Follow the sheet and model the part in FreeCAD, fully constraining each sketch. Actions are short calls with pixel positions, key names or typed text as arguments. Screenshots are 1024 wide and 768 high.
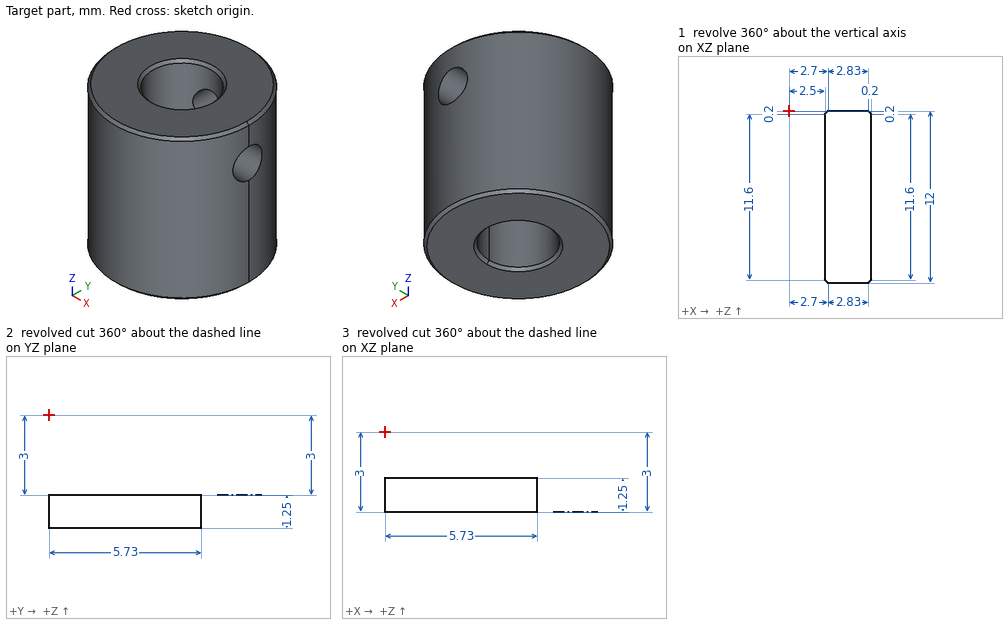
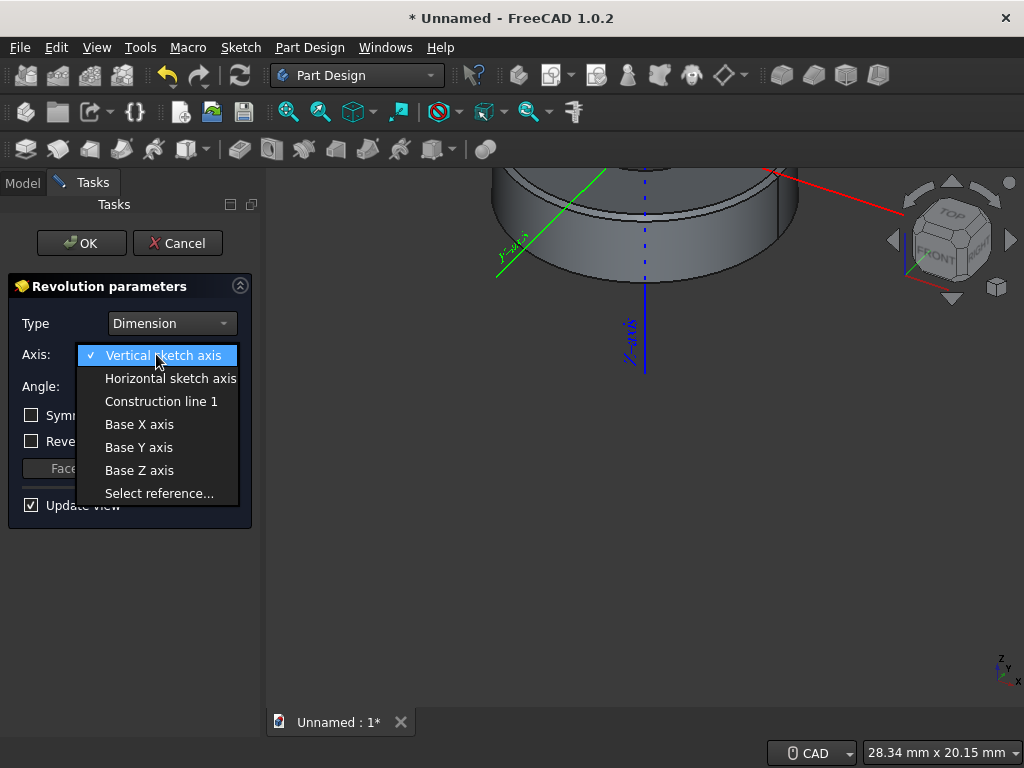
click(156, 402)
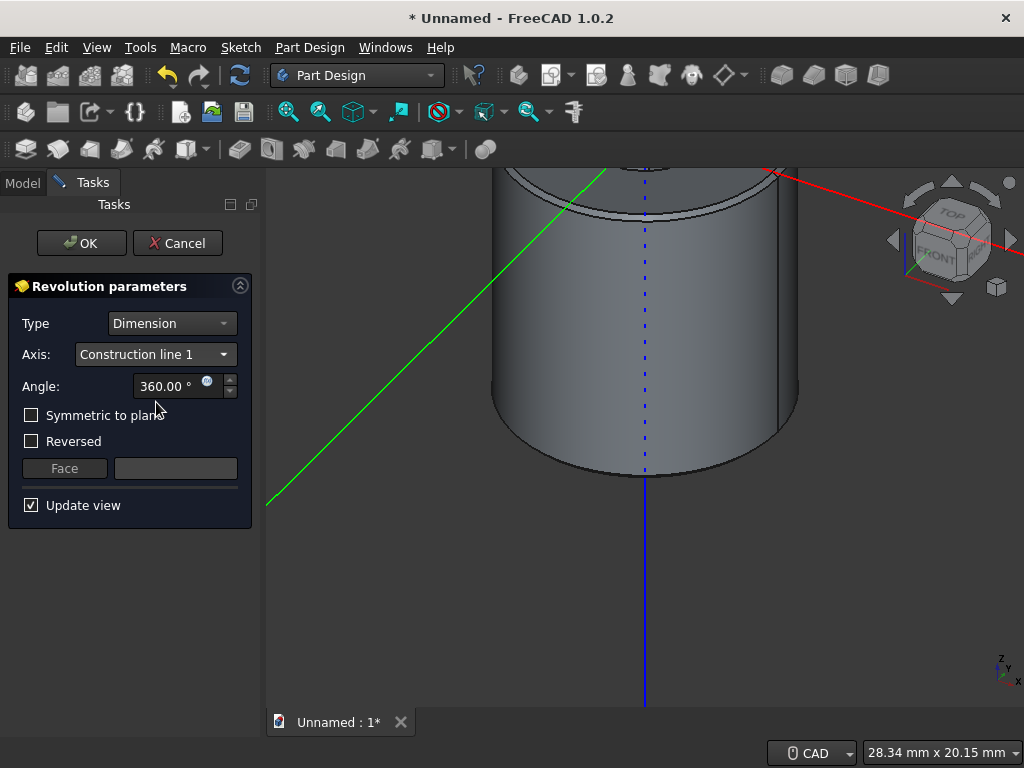
click(82, 243)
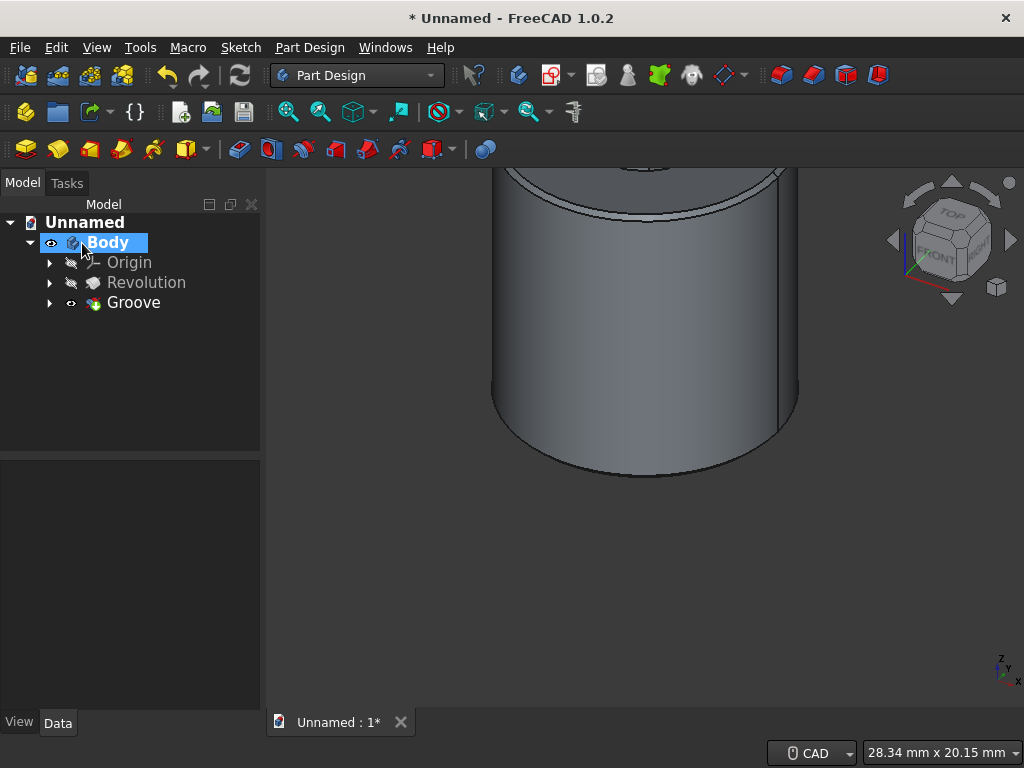
click(290, 112)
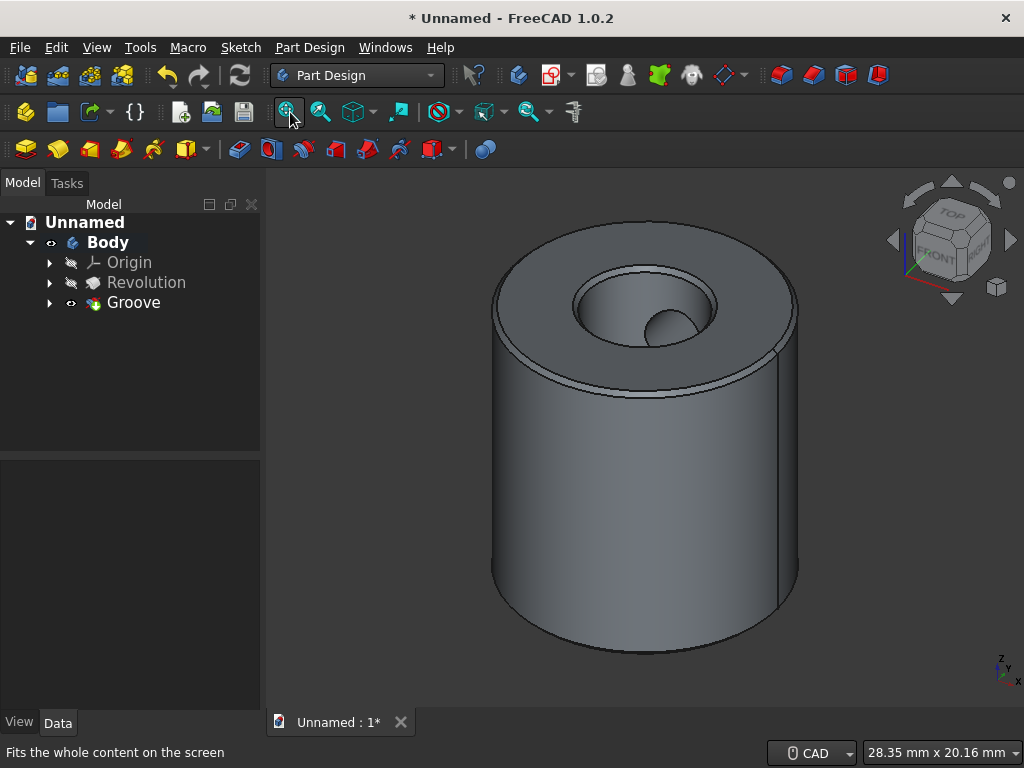
click(552, 76)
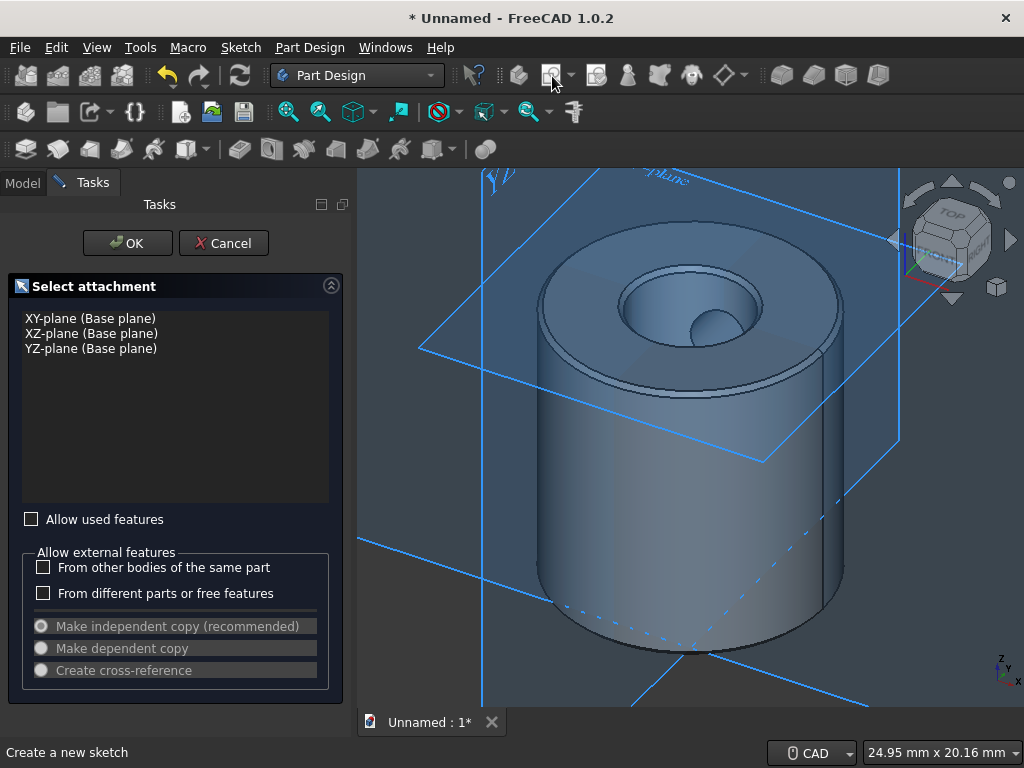
click(82, 334)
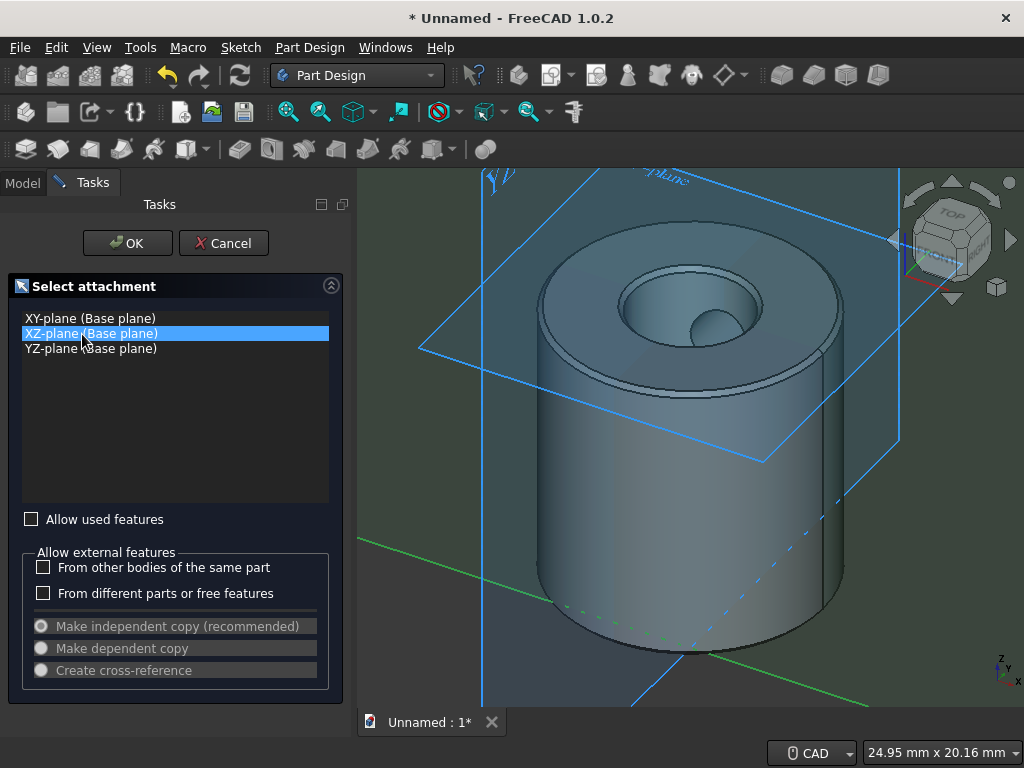
click(128, 243)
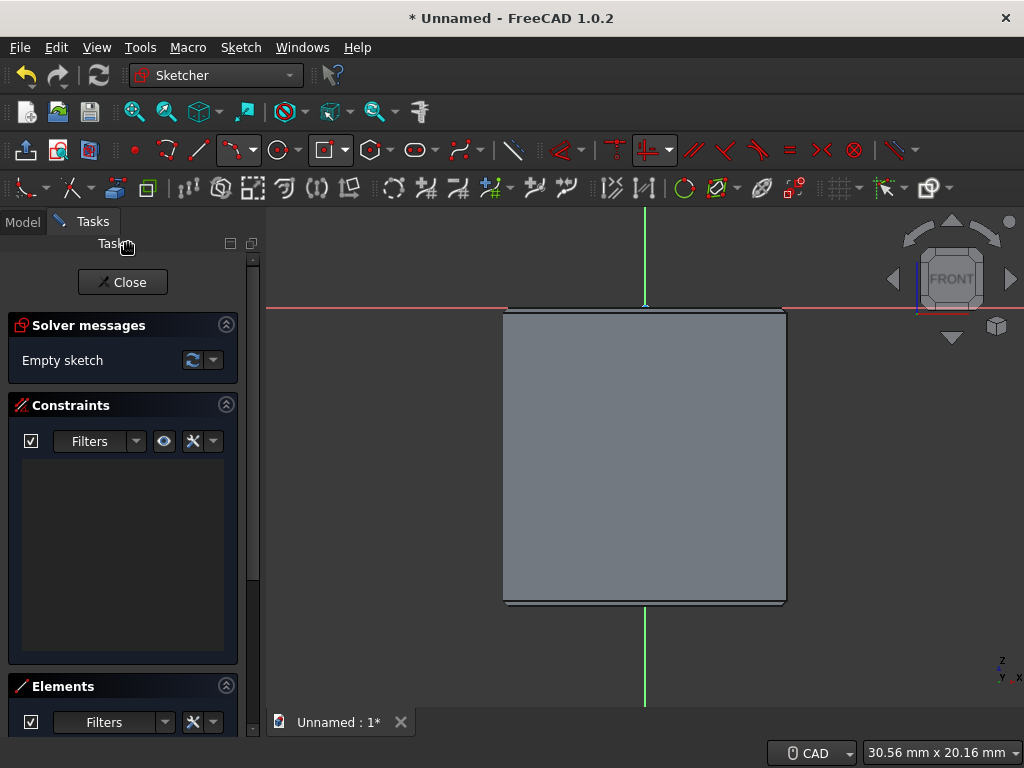
click(90, 150)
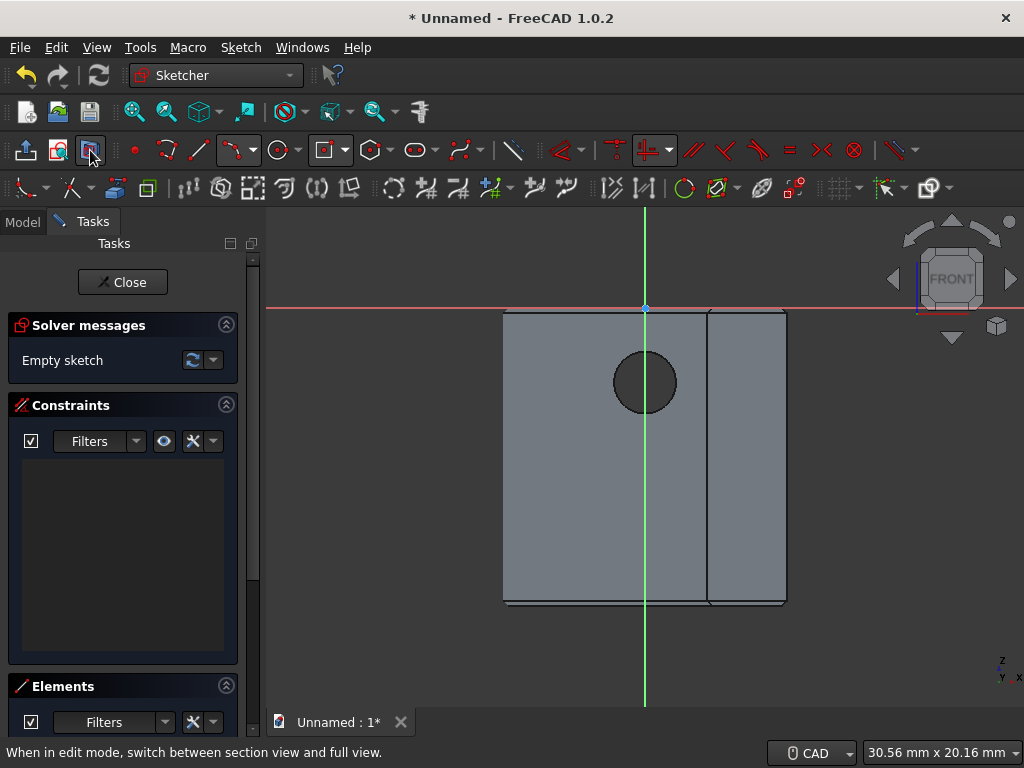
scroll(859, 235, up, 3)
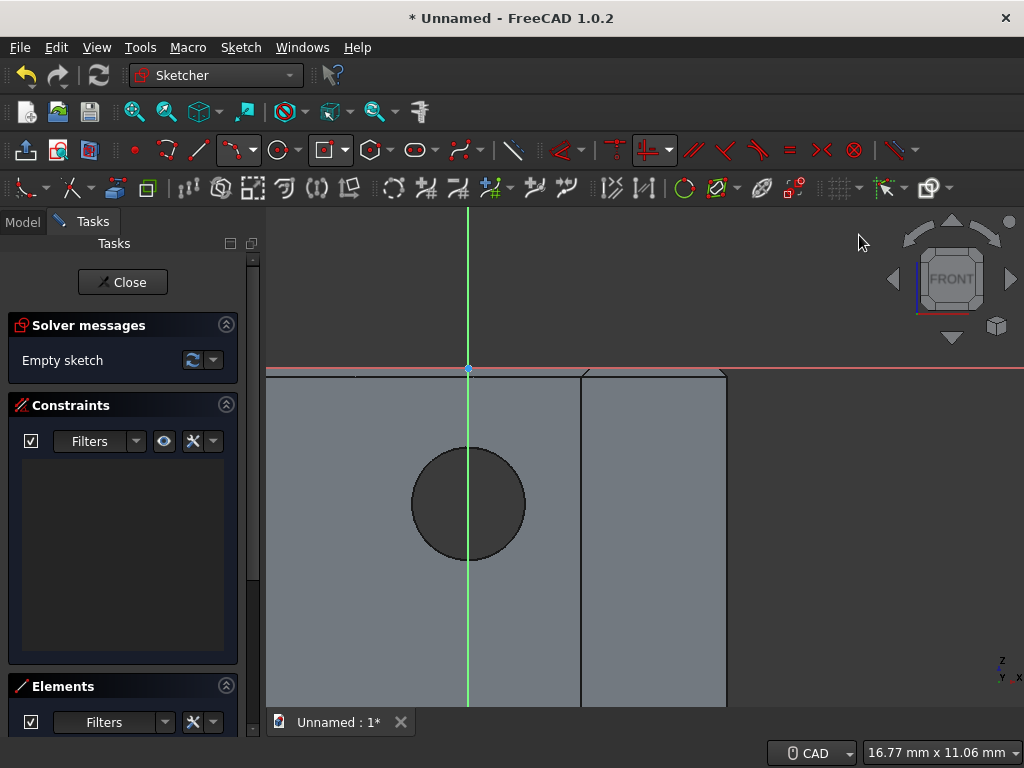
key(g)
key(r)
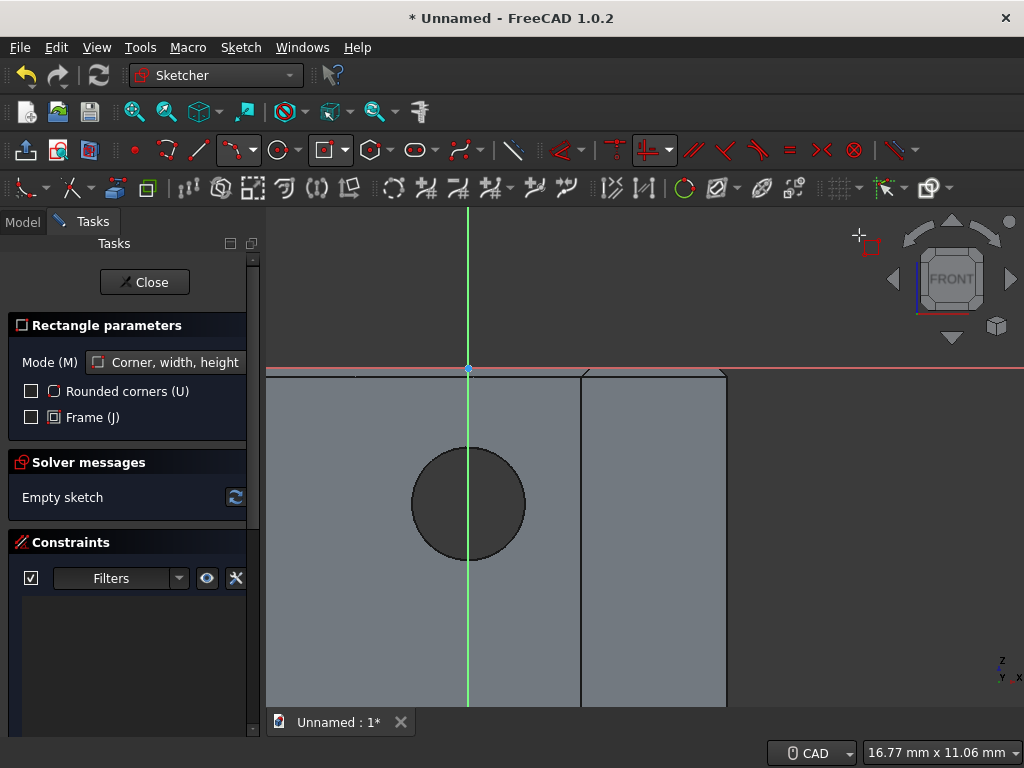
click(468, 447)
move(727, 504)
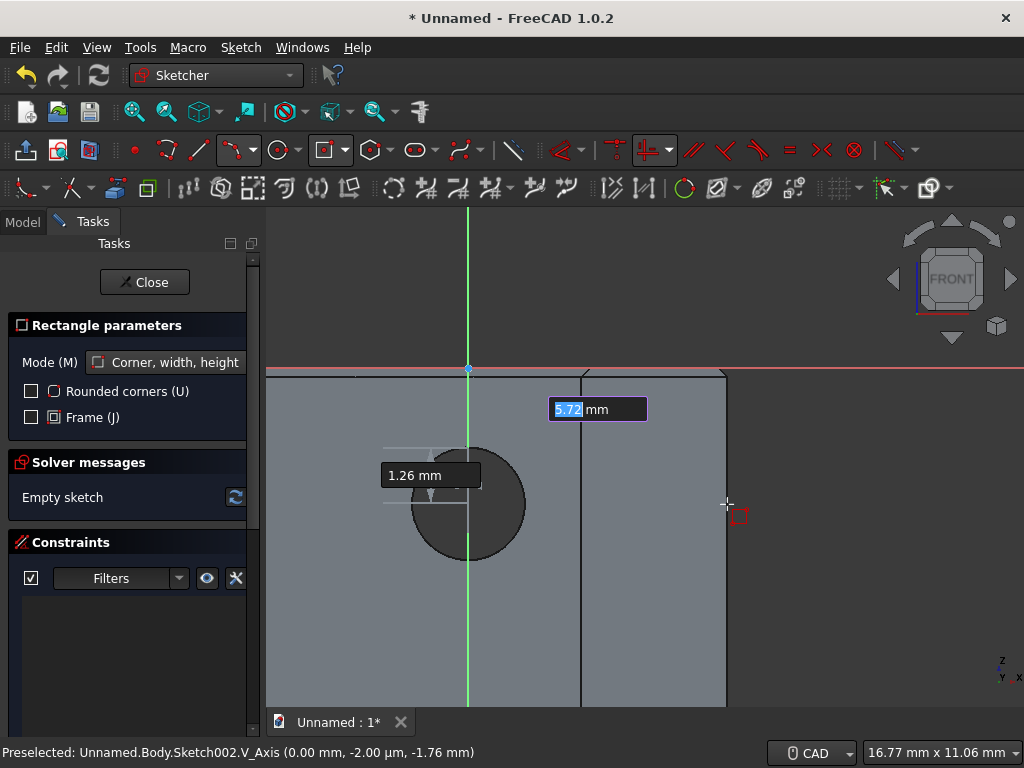
text(5.73)
key(Tab)
text(1.25)
key(Return)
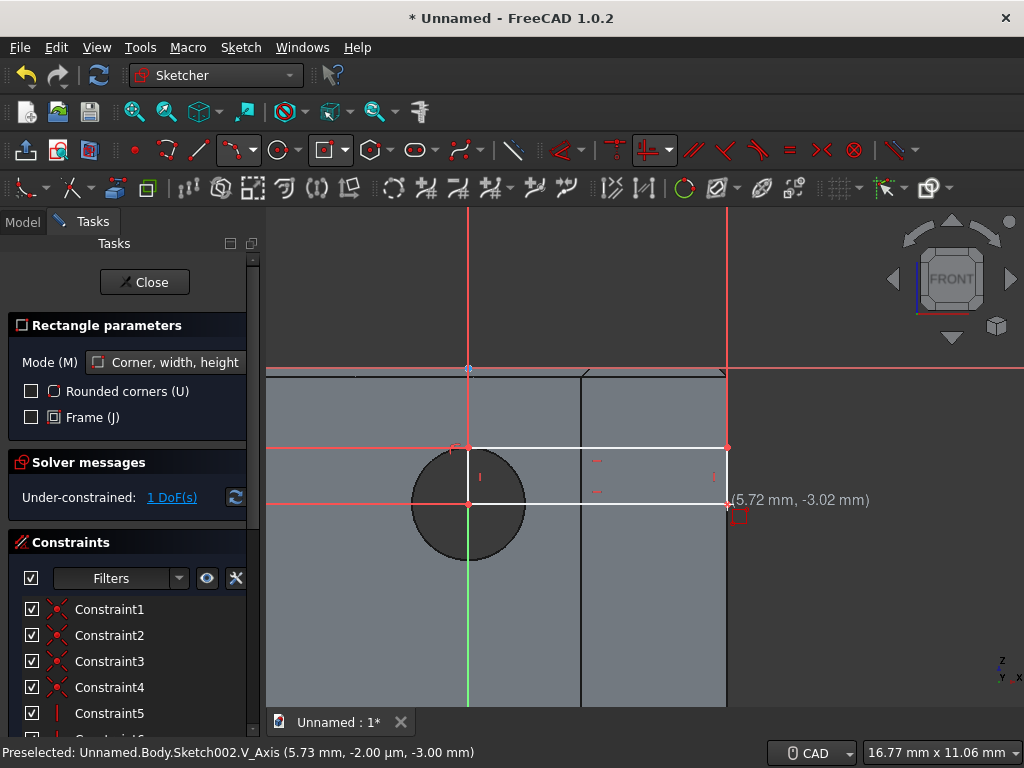
key(g)
key(l)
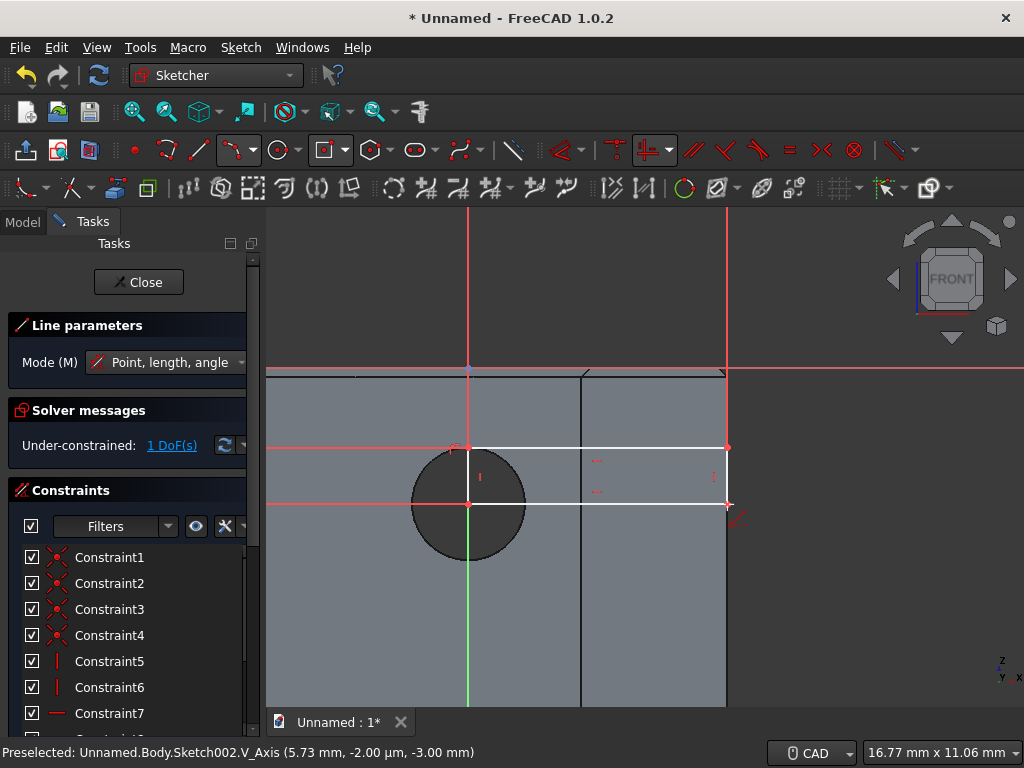
click(753, 504)
click(831, 504)
key(Escape)